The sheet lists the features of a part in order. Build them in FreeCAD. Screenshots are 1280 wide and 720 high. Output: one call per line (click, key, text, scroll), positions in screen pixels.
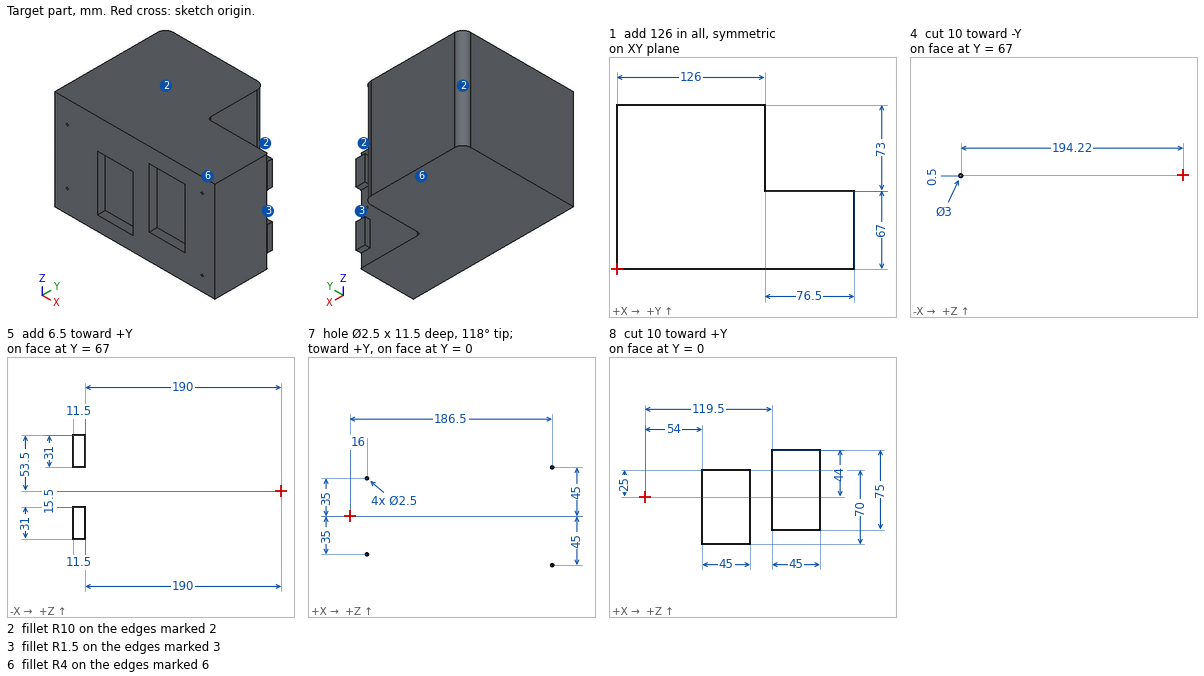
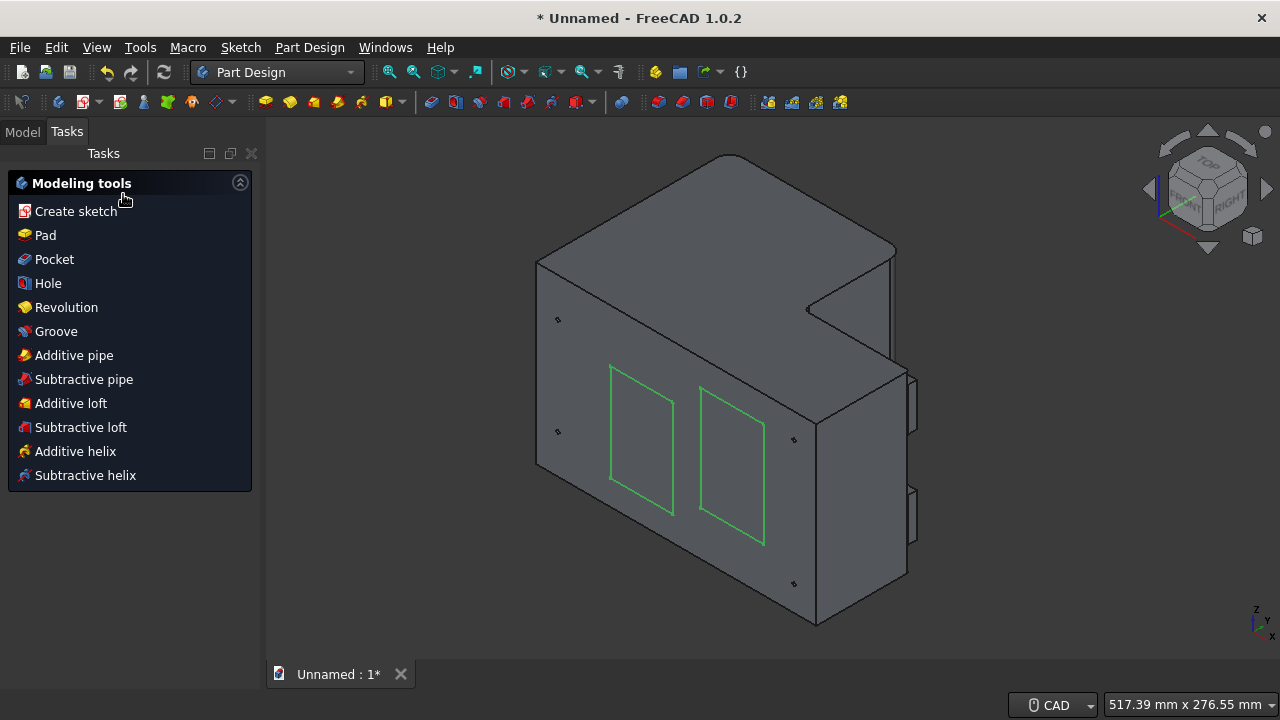
click(432, 102)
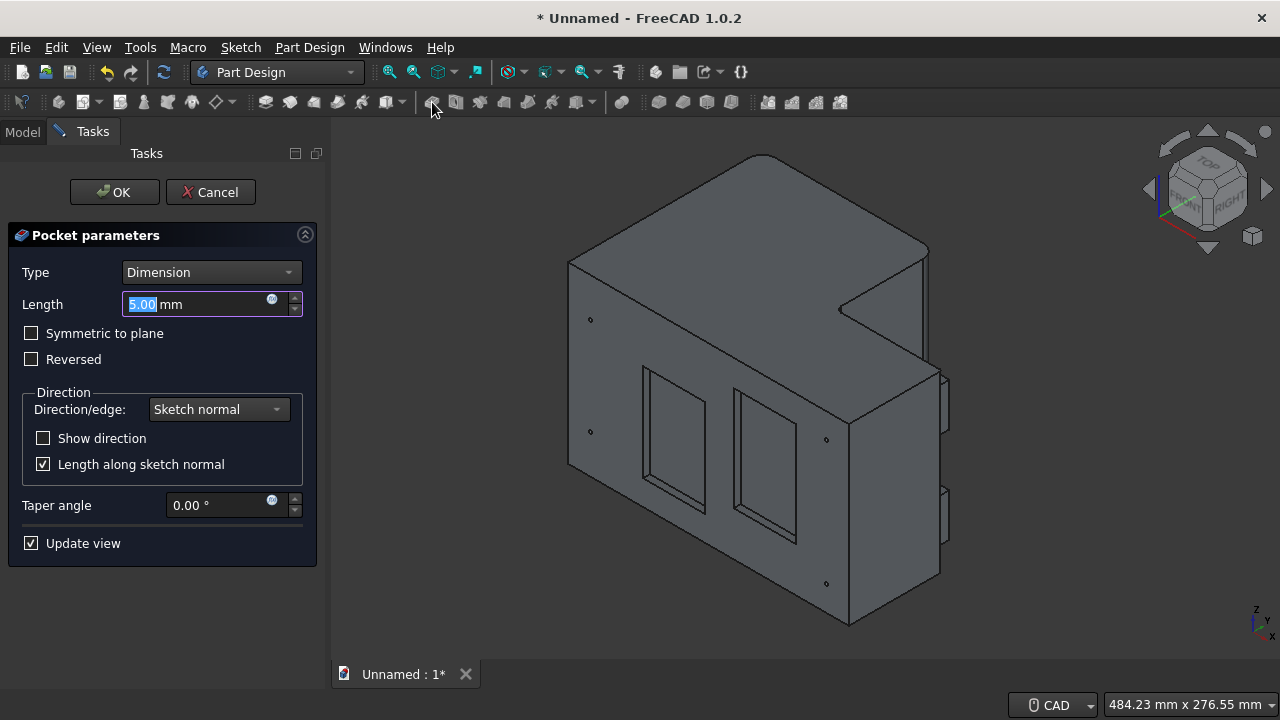
text(10)
key(Tab)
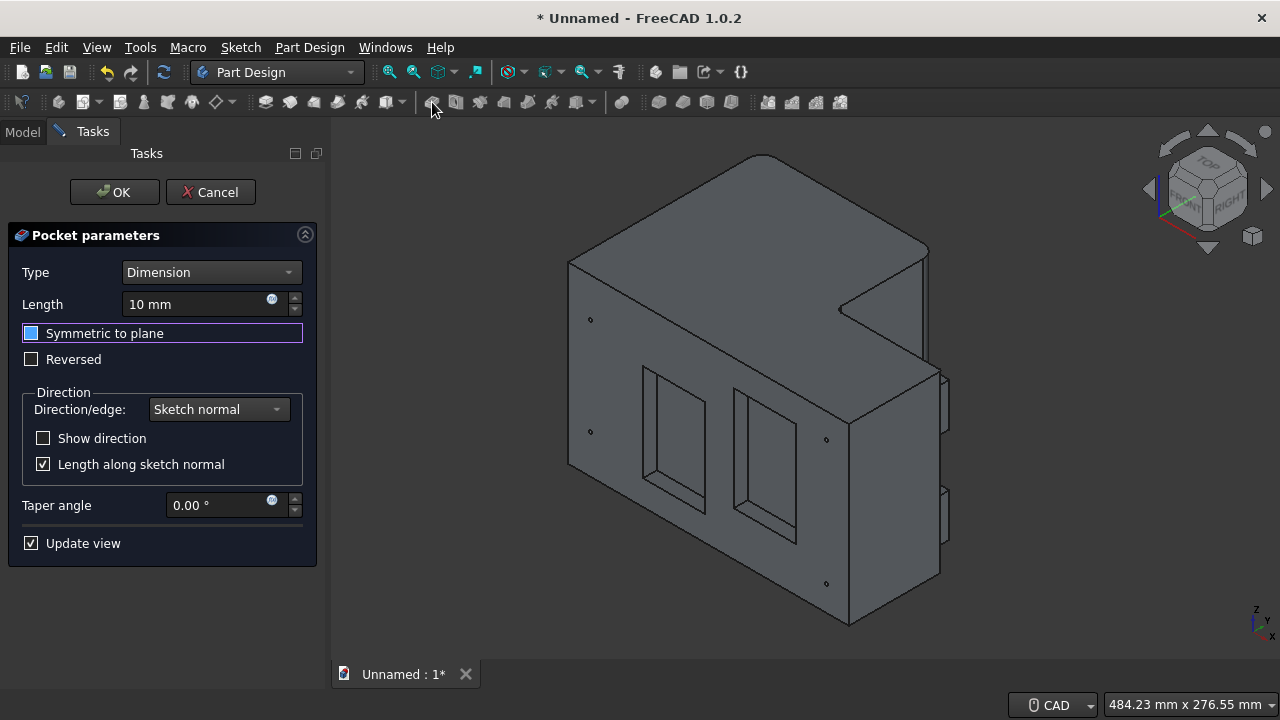
click(115, 192)